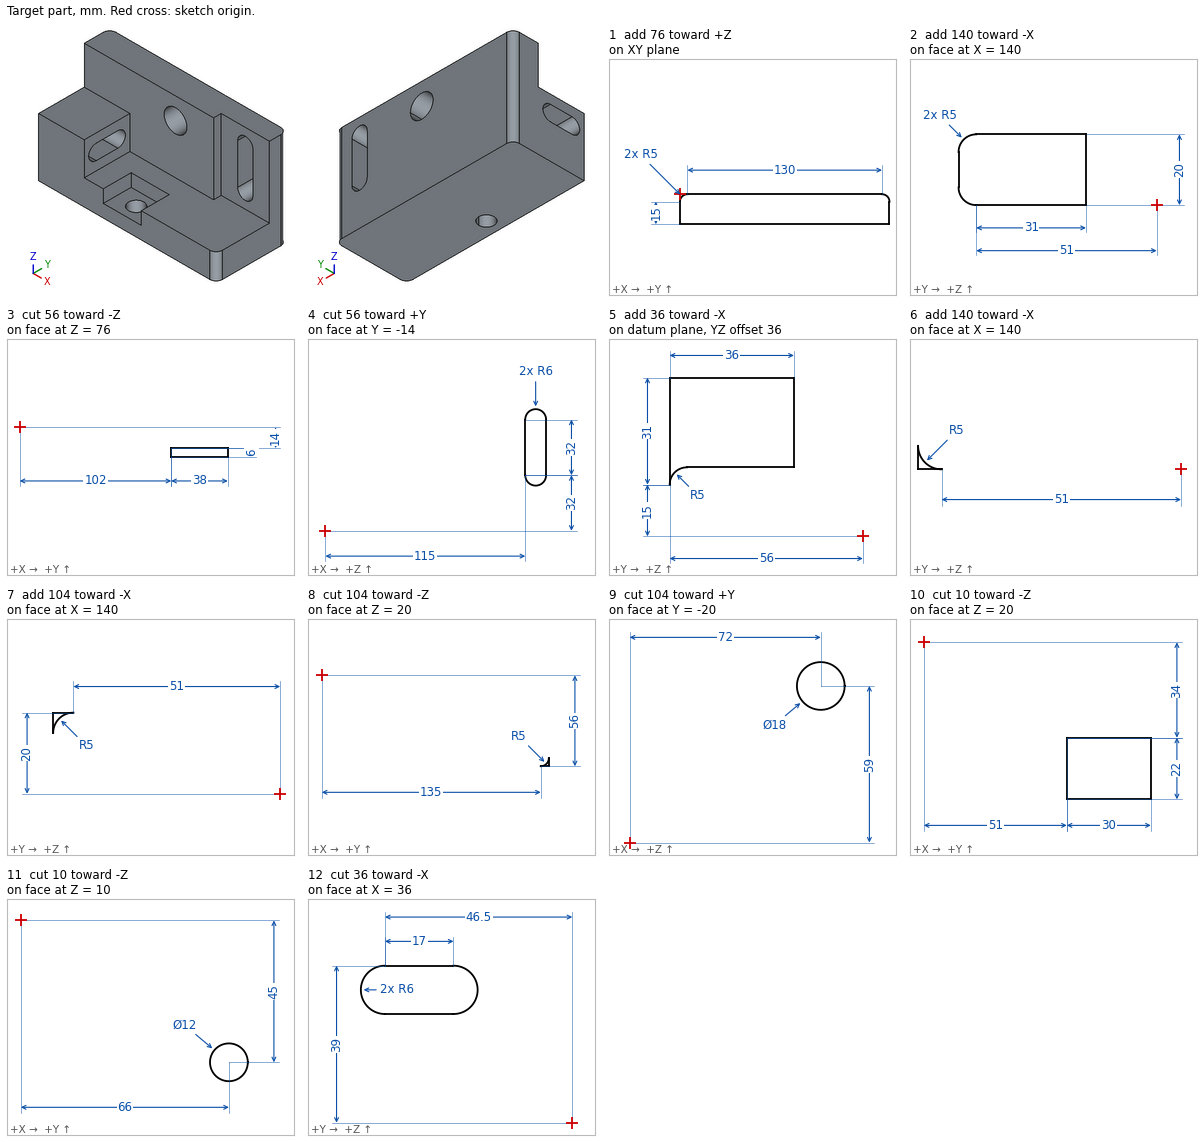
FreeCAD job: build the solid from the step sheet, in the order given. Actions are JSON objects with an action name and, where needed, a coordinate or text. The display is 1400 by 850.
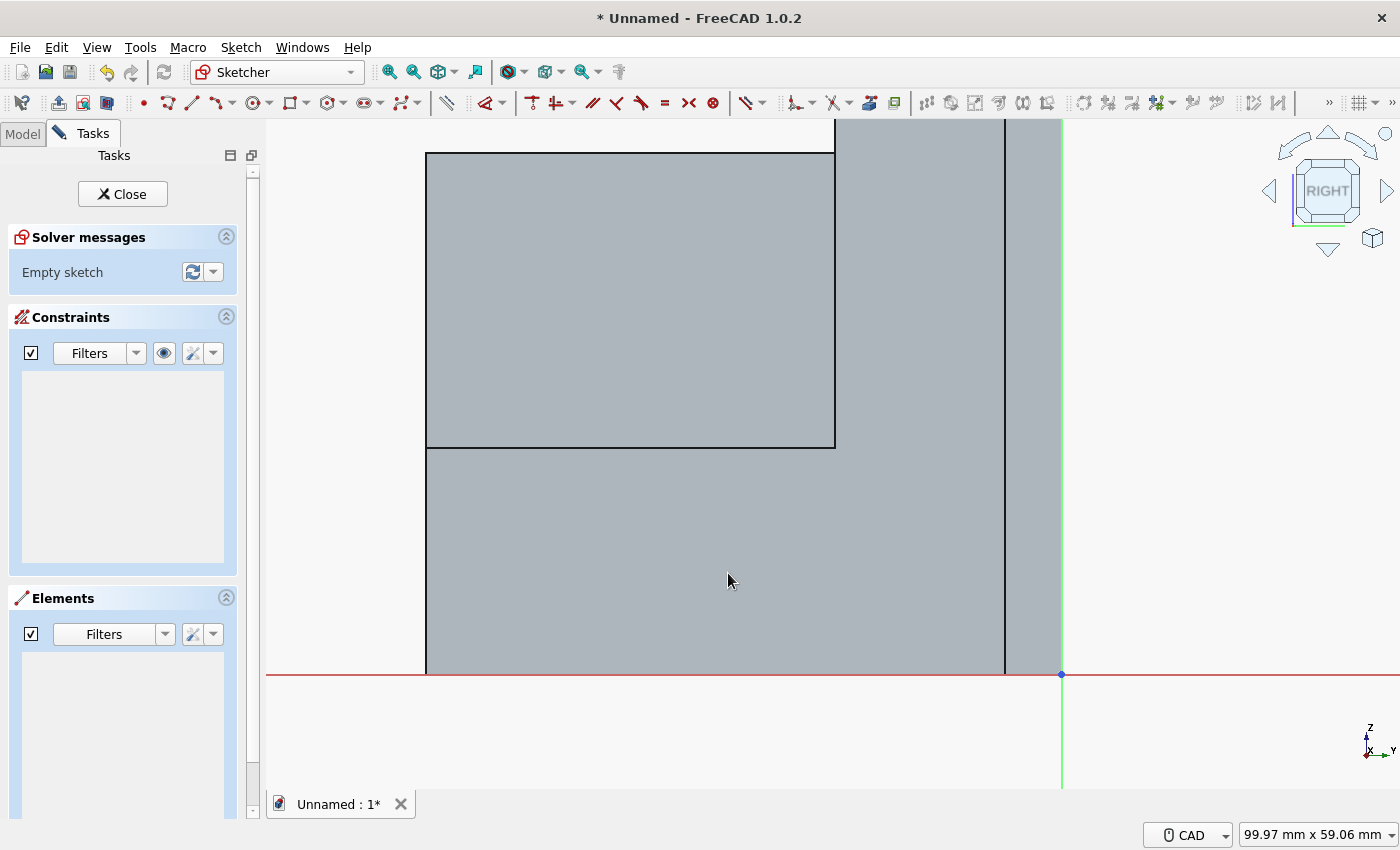
{"action": "left_click", "coordinate": [364, 104]}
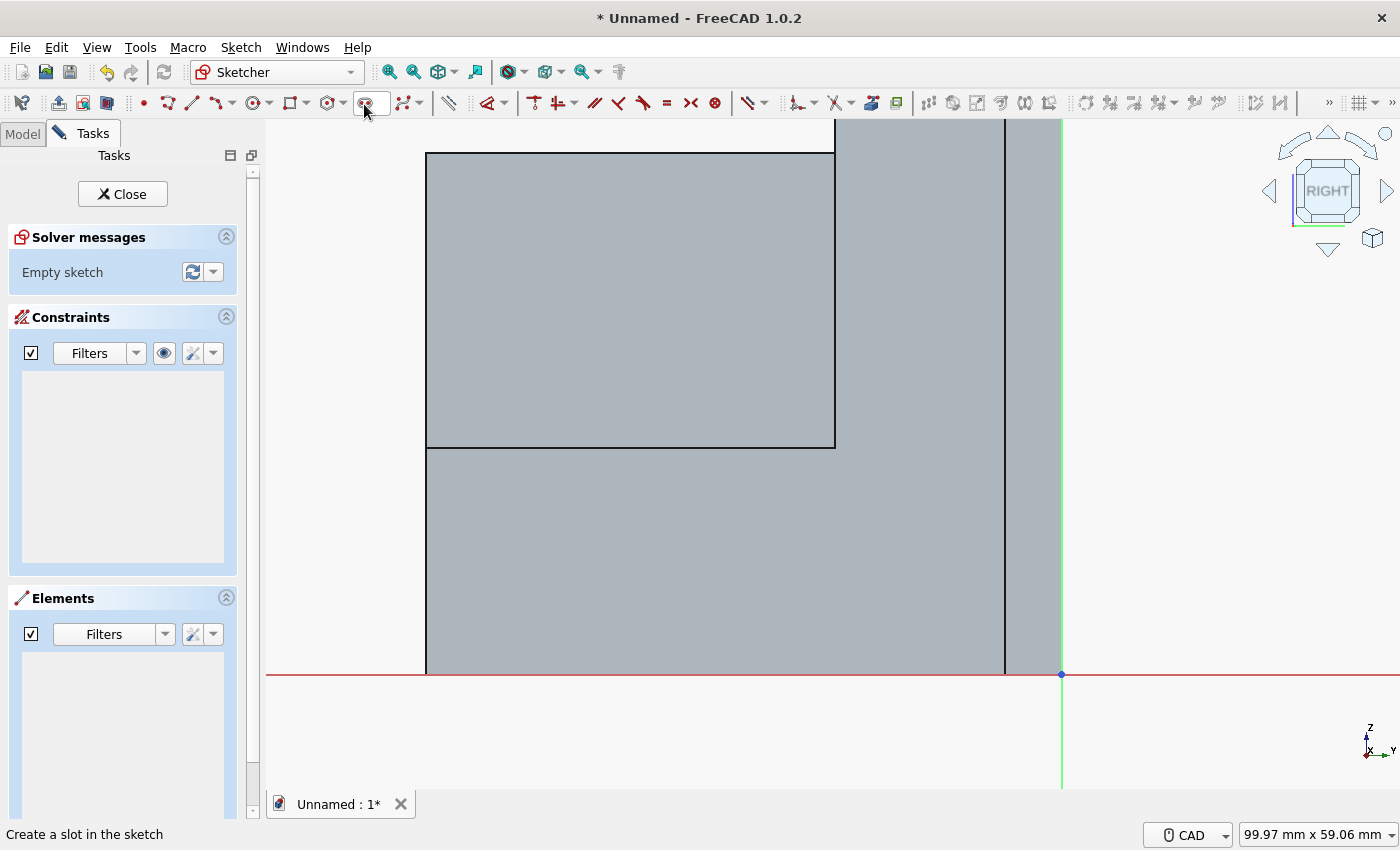
{"action": "left_click", "coordinate": [534, 300]}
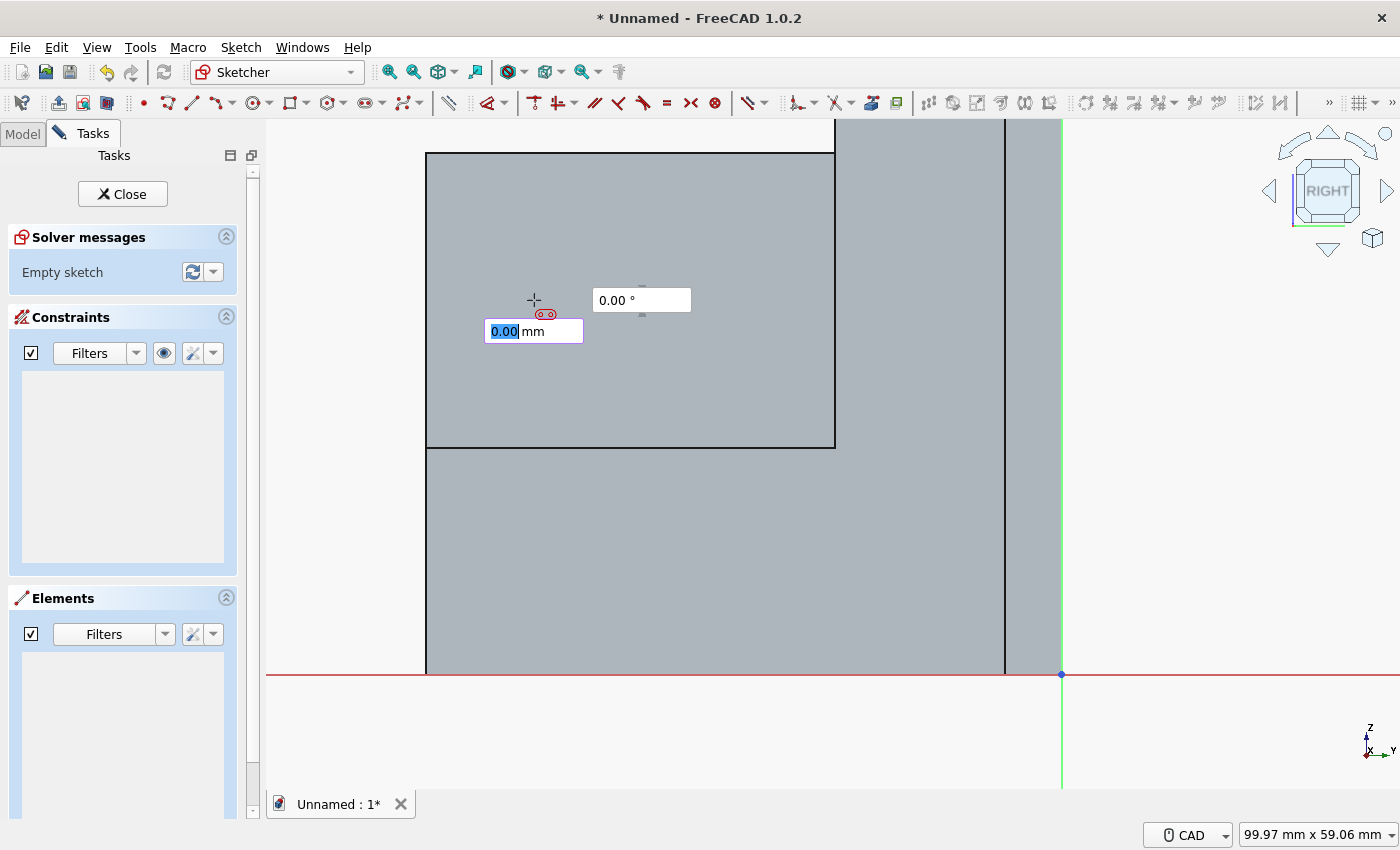
{"action": "left_click", "coordinate": [727, 300]}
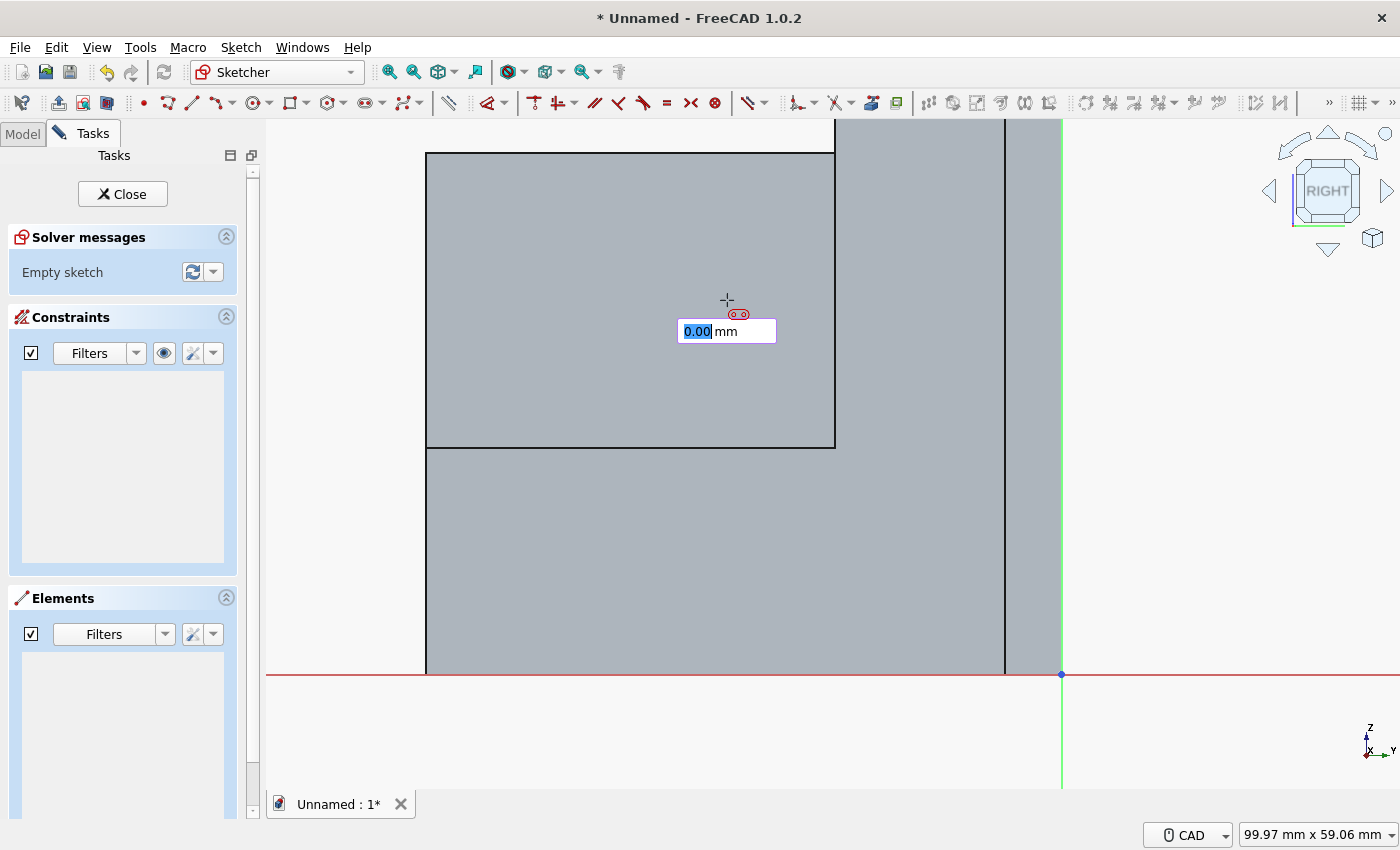
{"action": "left_click", "coordinate": [630, 232]}
{"action": "key", "text": "Escape"}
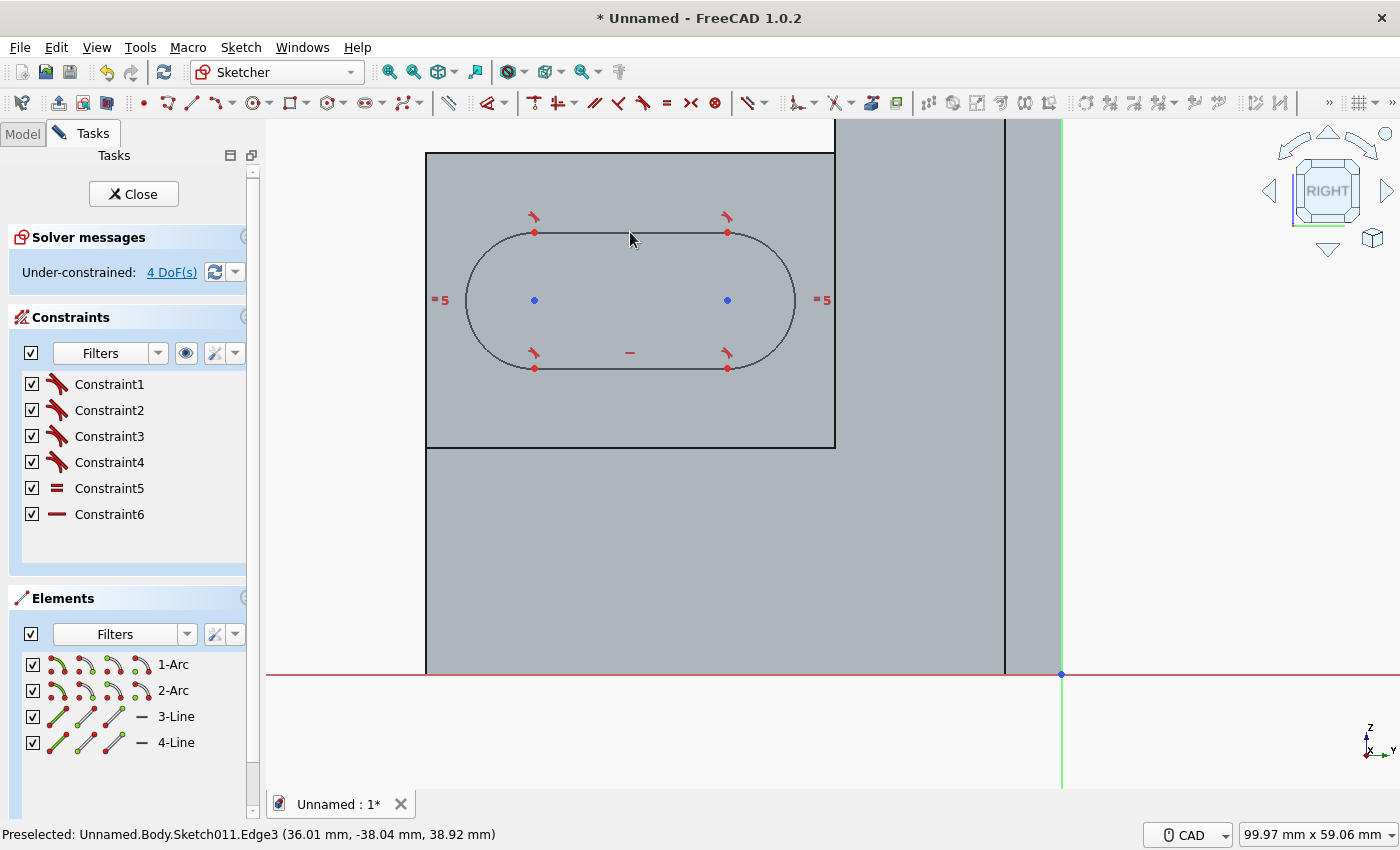
{"action": "key", "text": "d"}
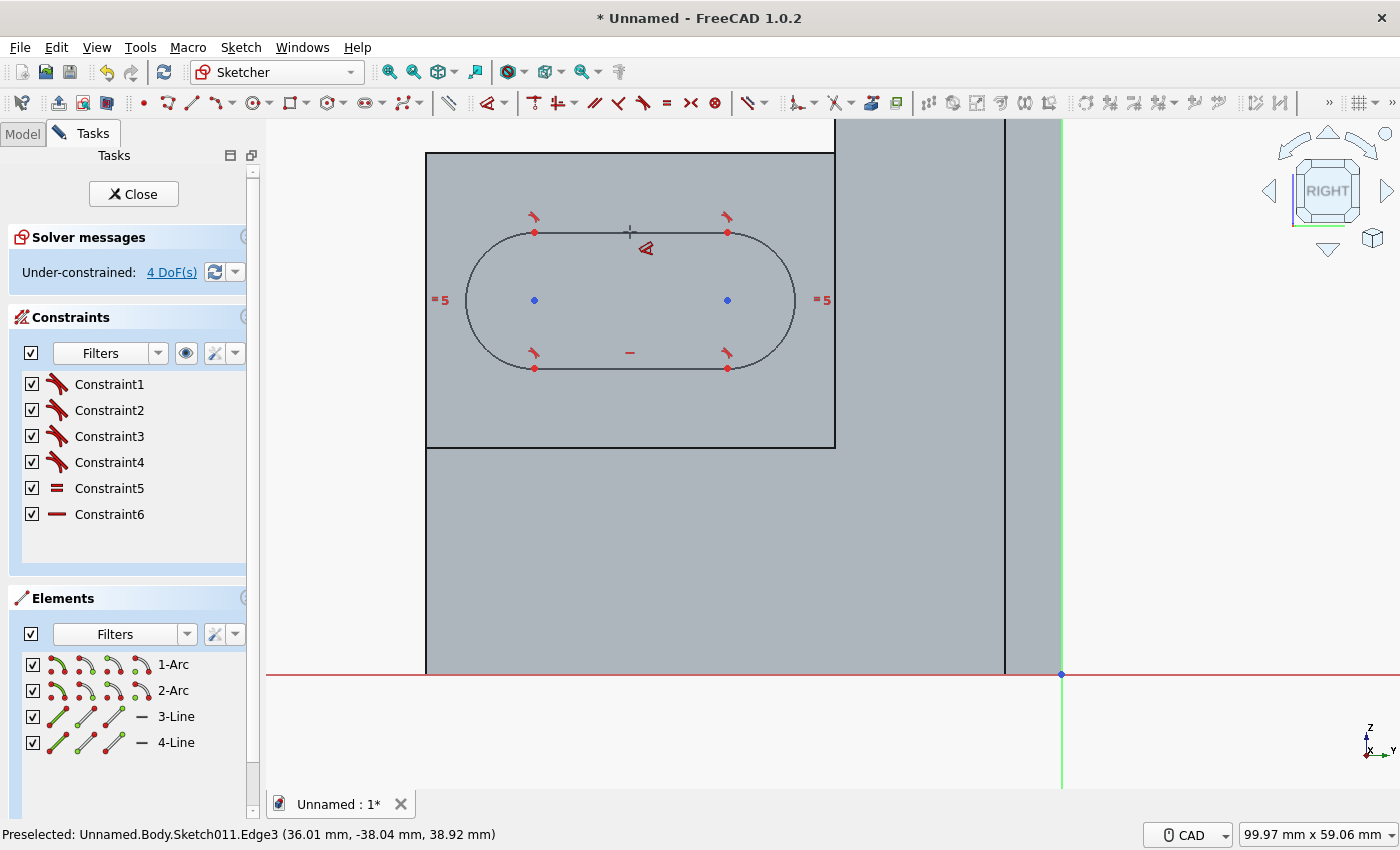
{"action": "left_click", "coordinate": [479, 261]}
{"action": "left_click", "coordinate": [453, 242]}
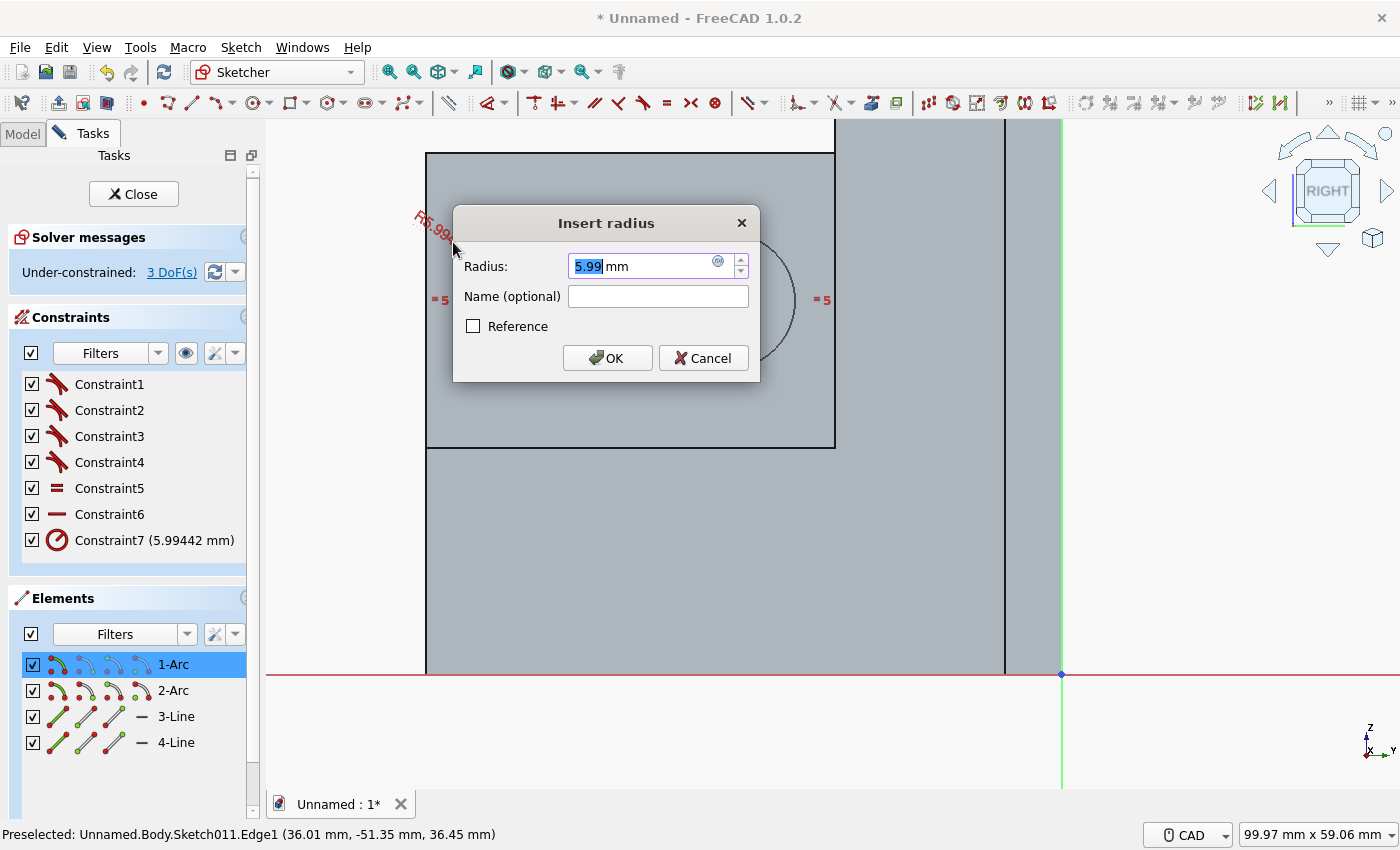
{"action": "type", "text": "6"}
{"action": "key", "text": "Return"}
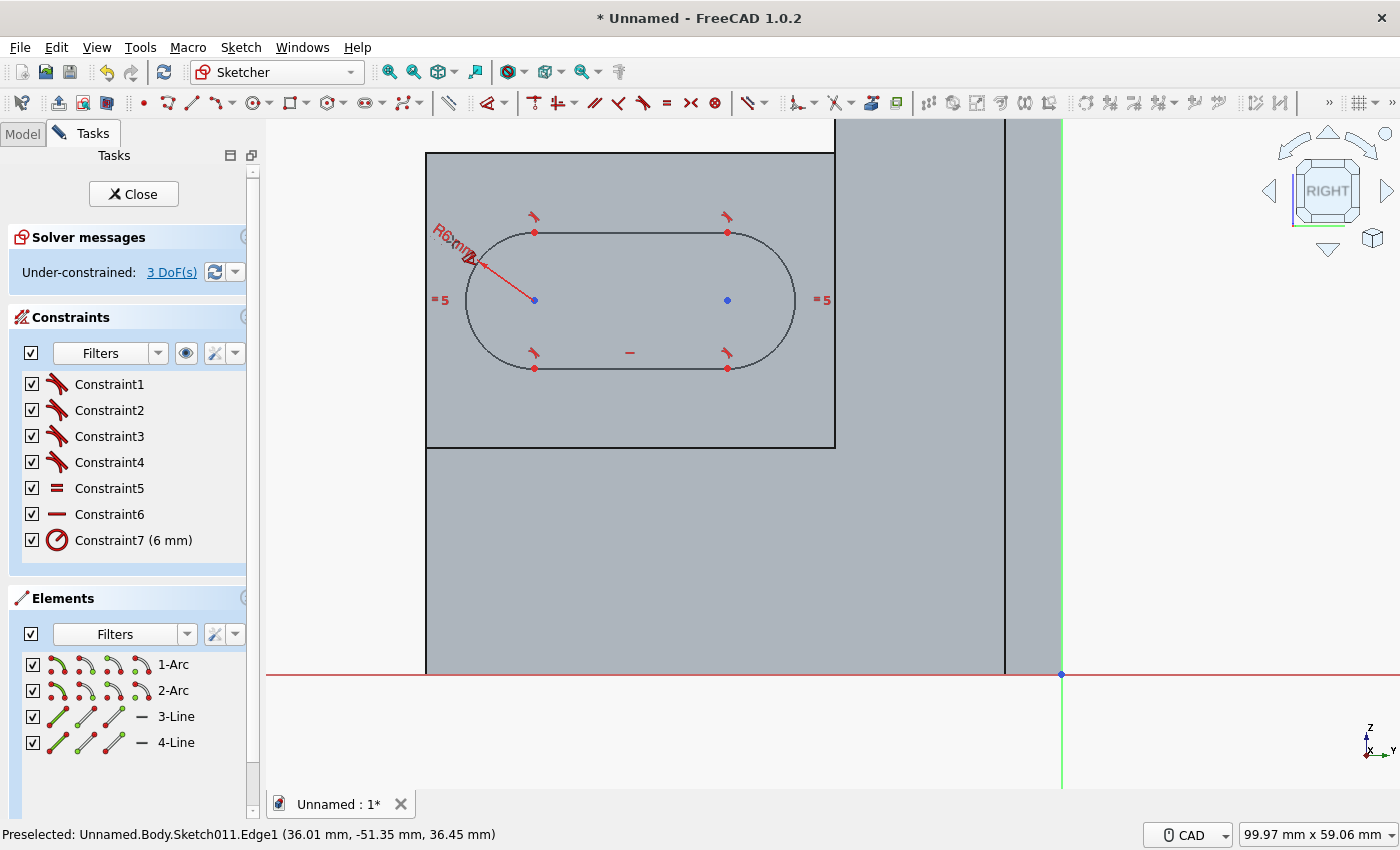
{"action": "left_click", "coordinate": [592, 233]}
{"action": "left_click", "coordinate": [631, 199]}